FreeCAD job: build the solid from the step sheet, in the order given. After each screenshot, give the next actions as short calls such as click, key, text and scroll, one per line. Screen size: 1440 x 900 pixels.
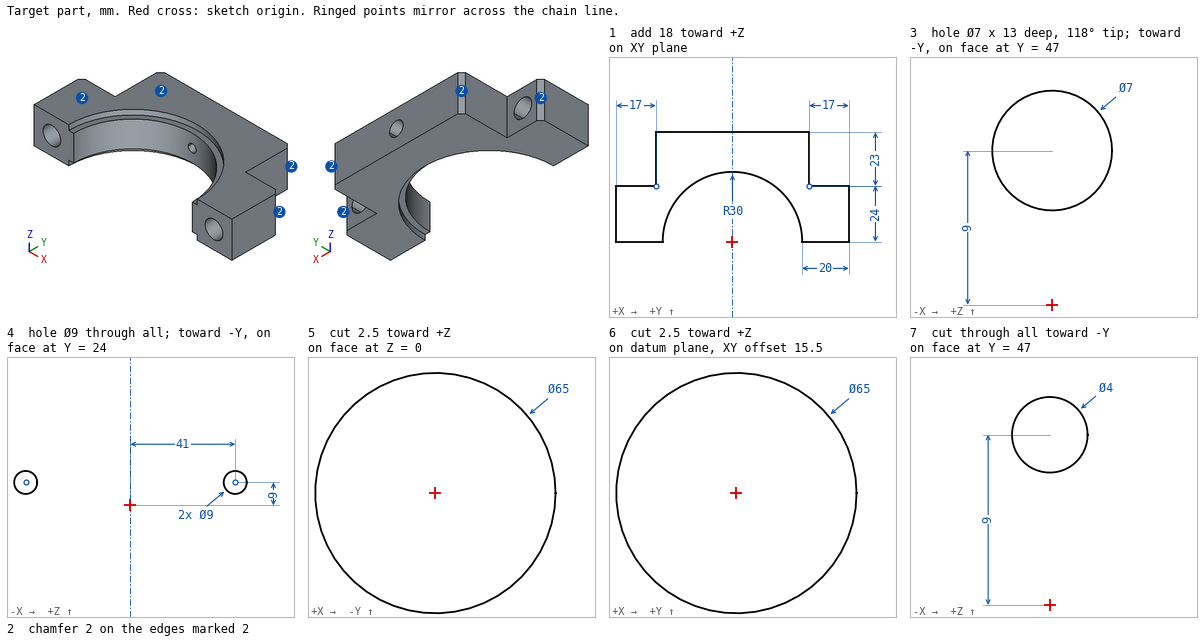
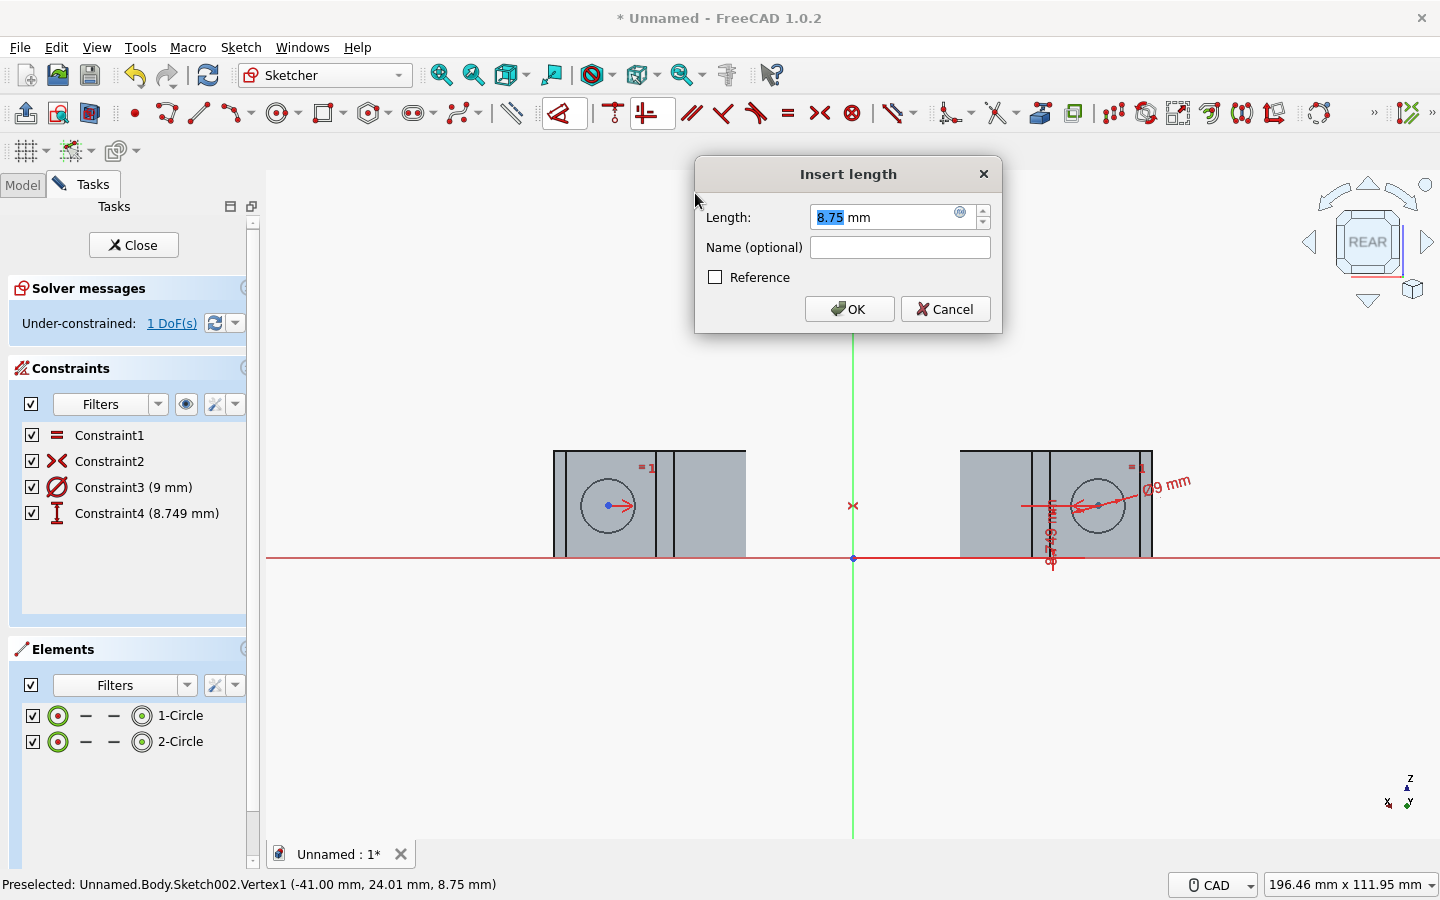
text(9)
key(Return)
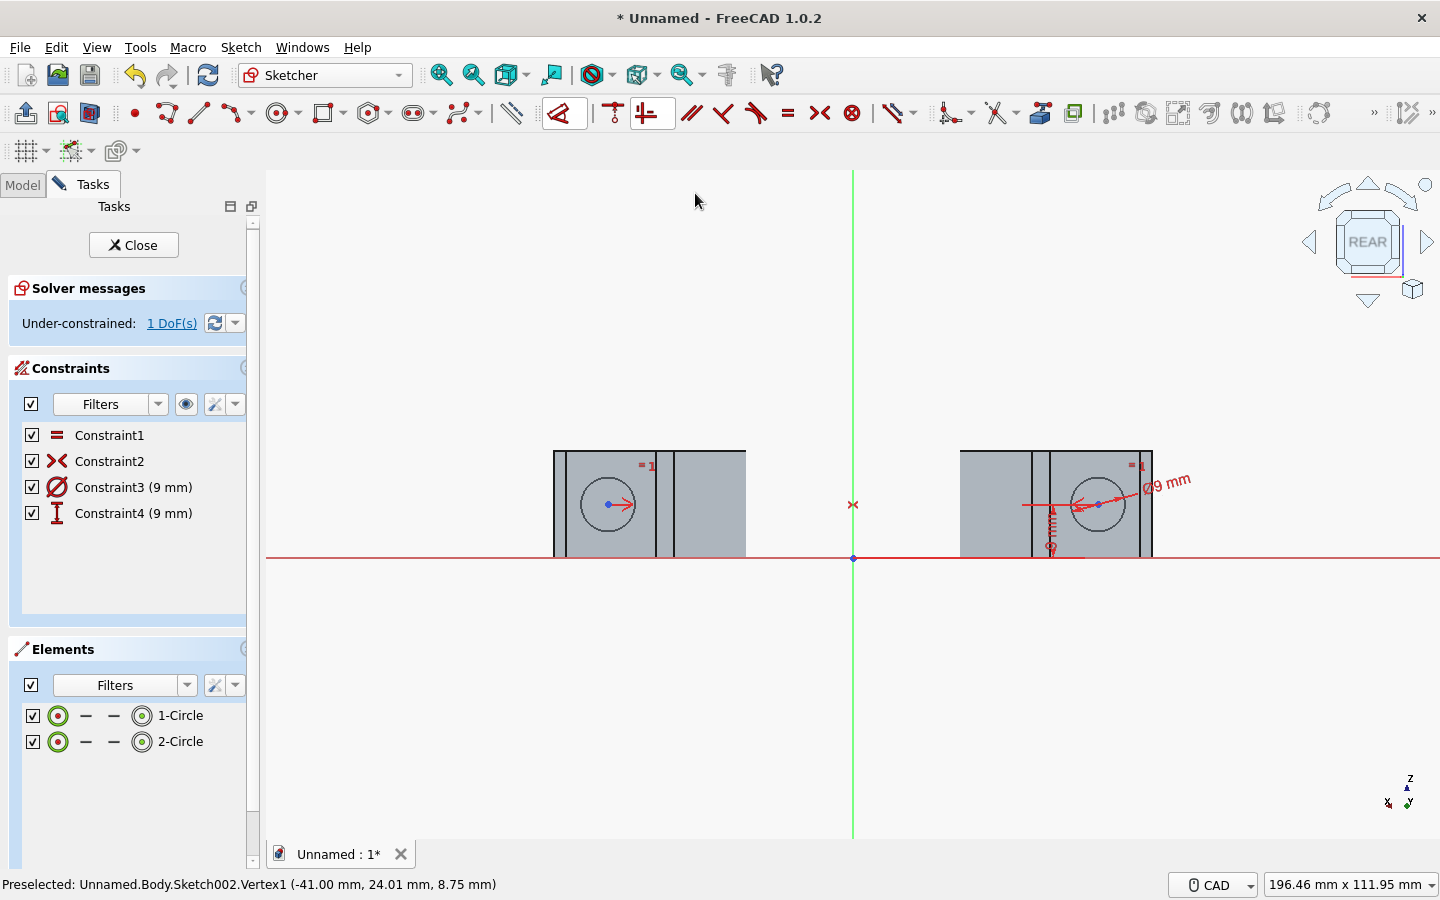
click(1098, 505)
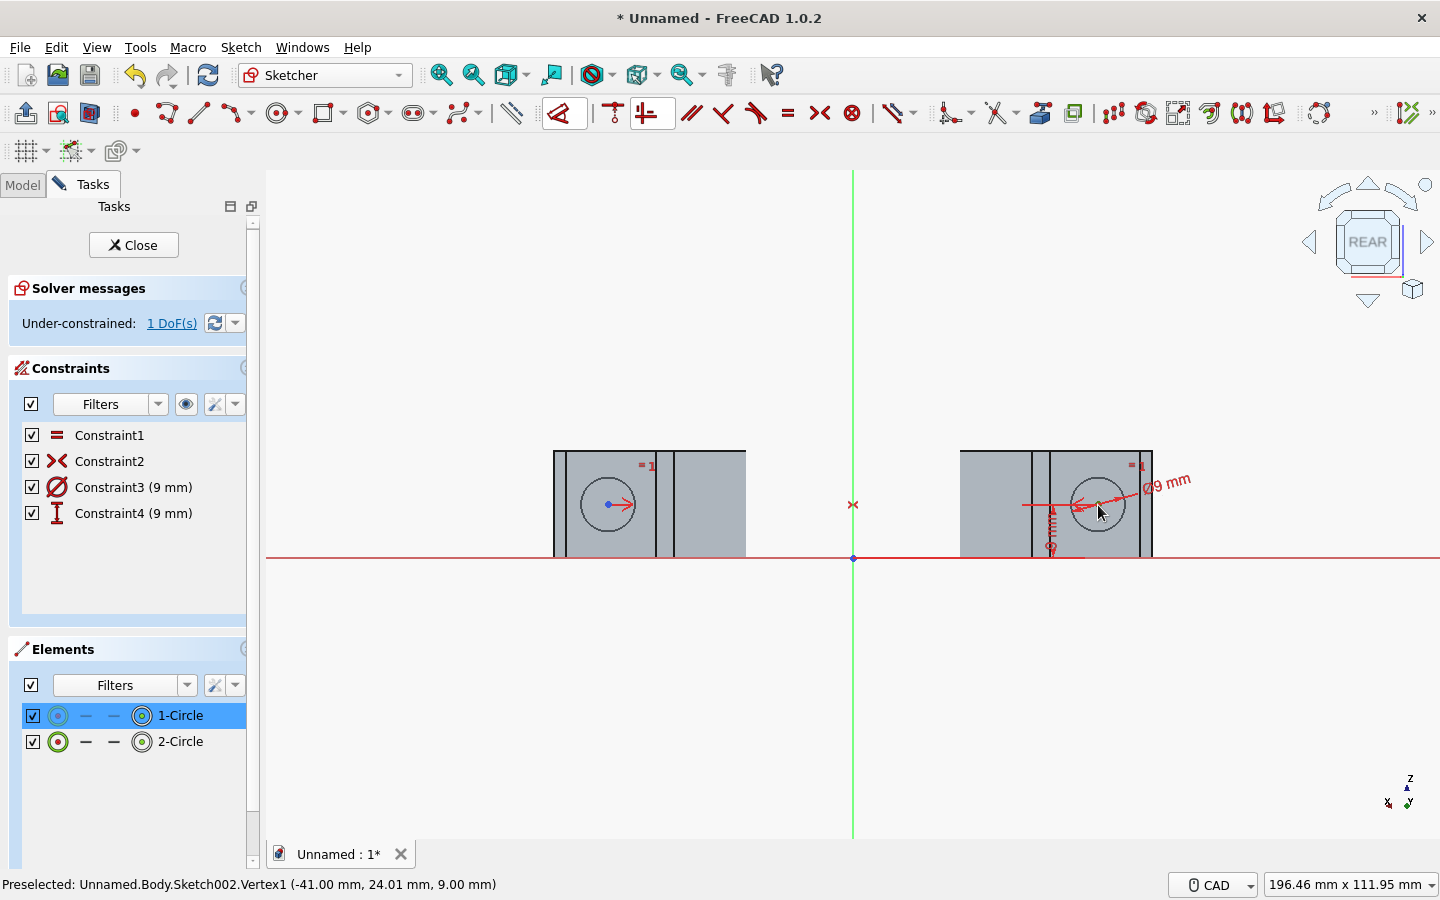
key(l)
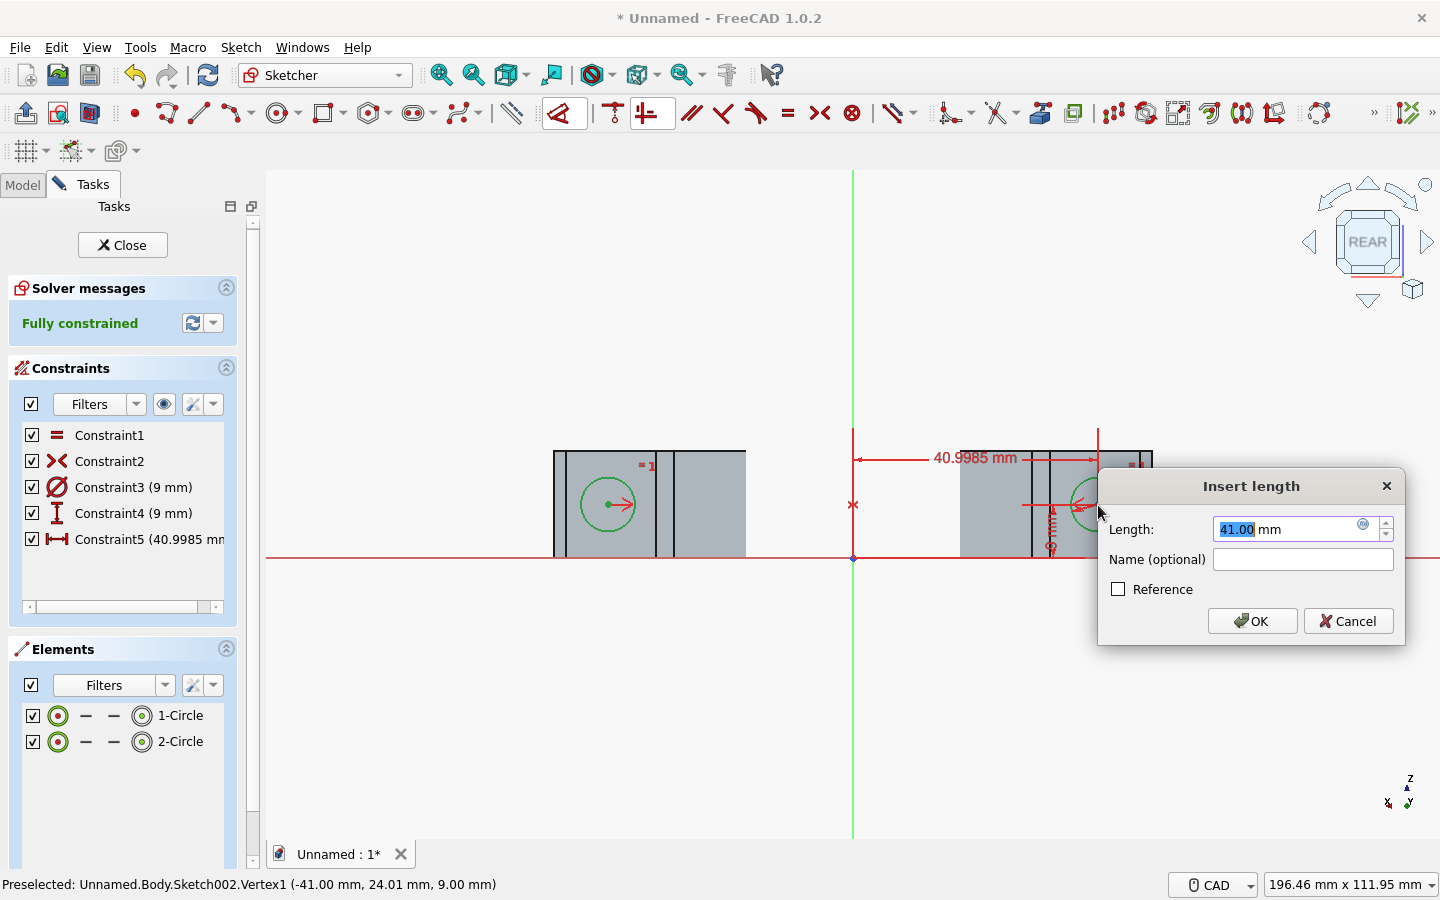
text(41)
key(Return)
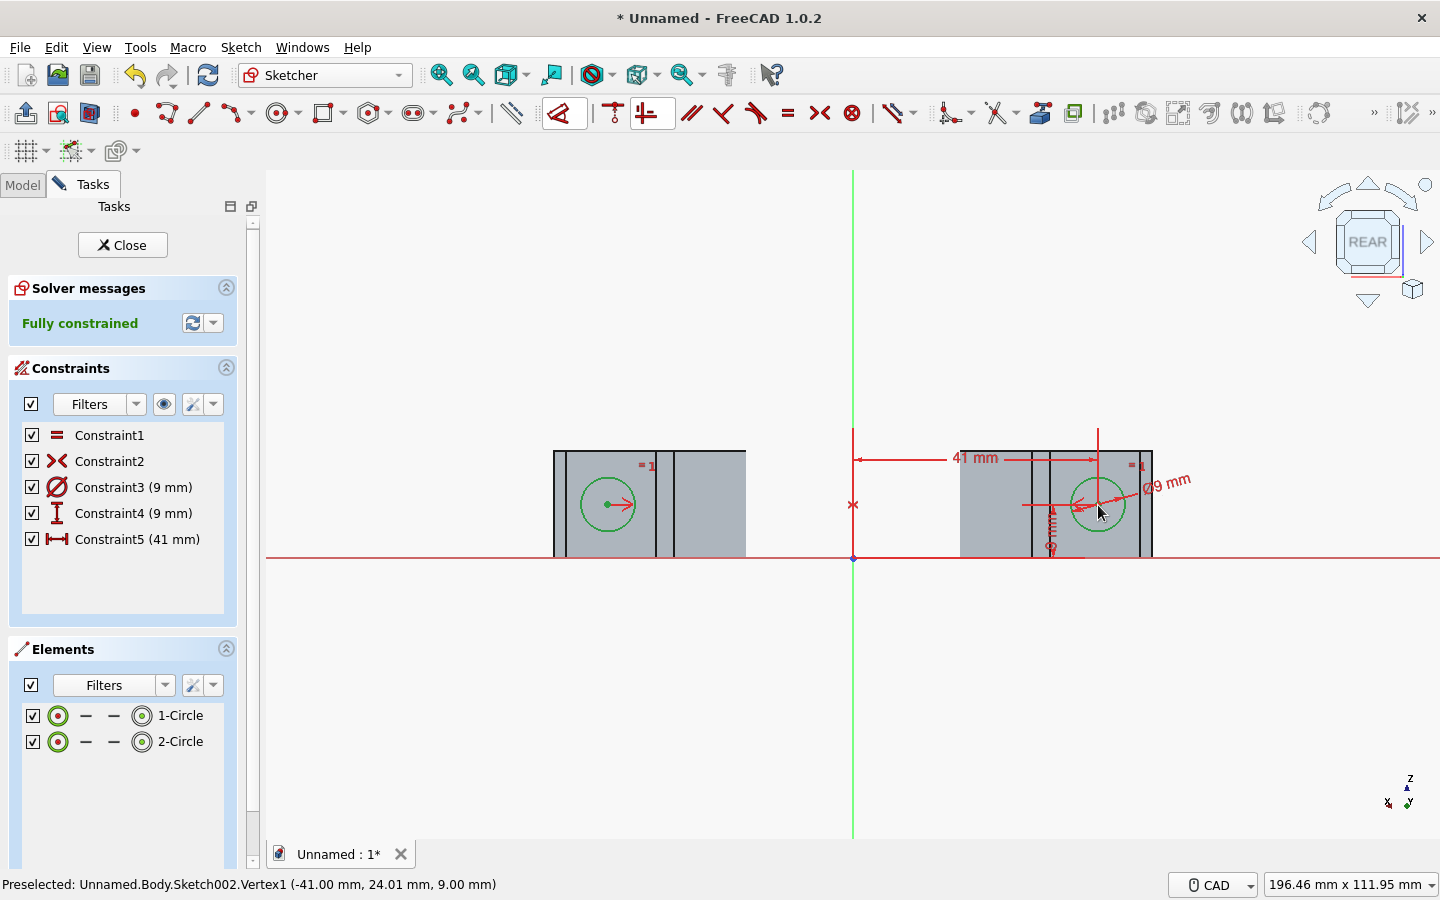
click(123, 245)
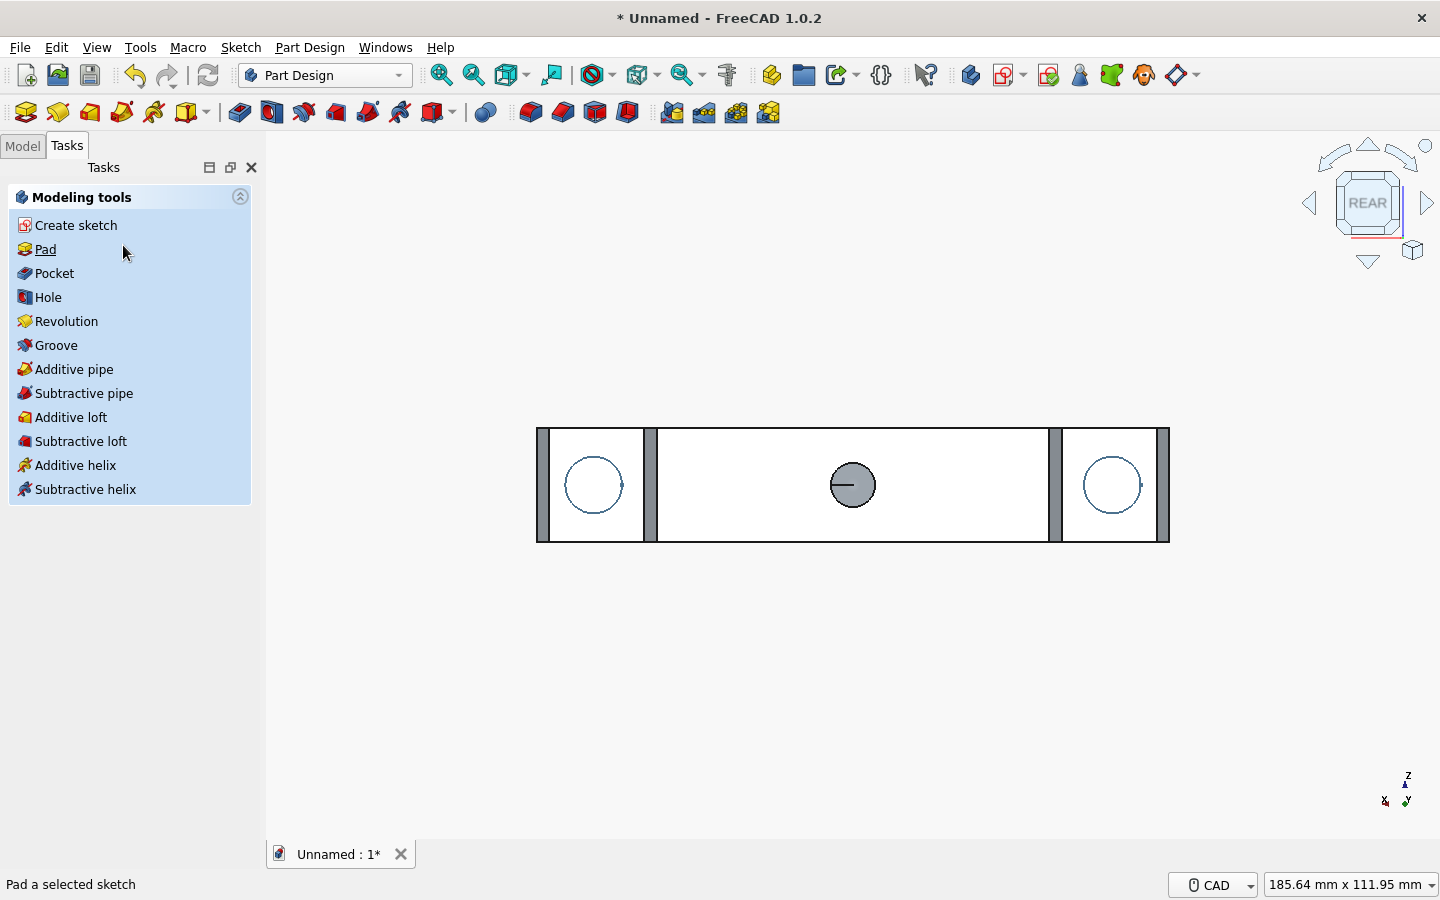
click(272, 112)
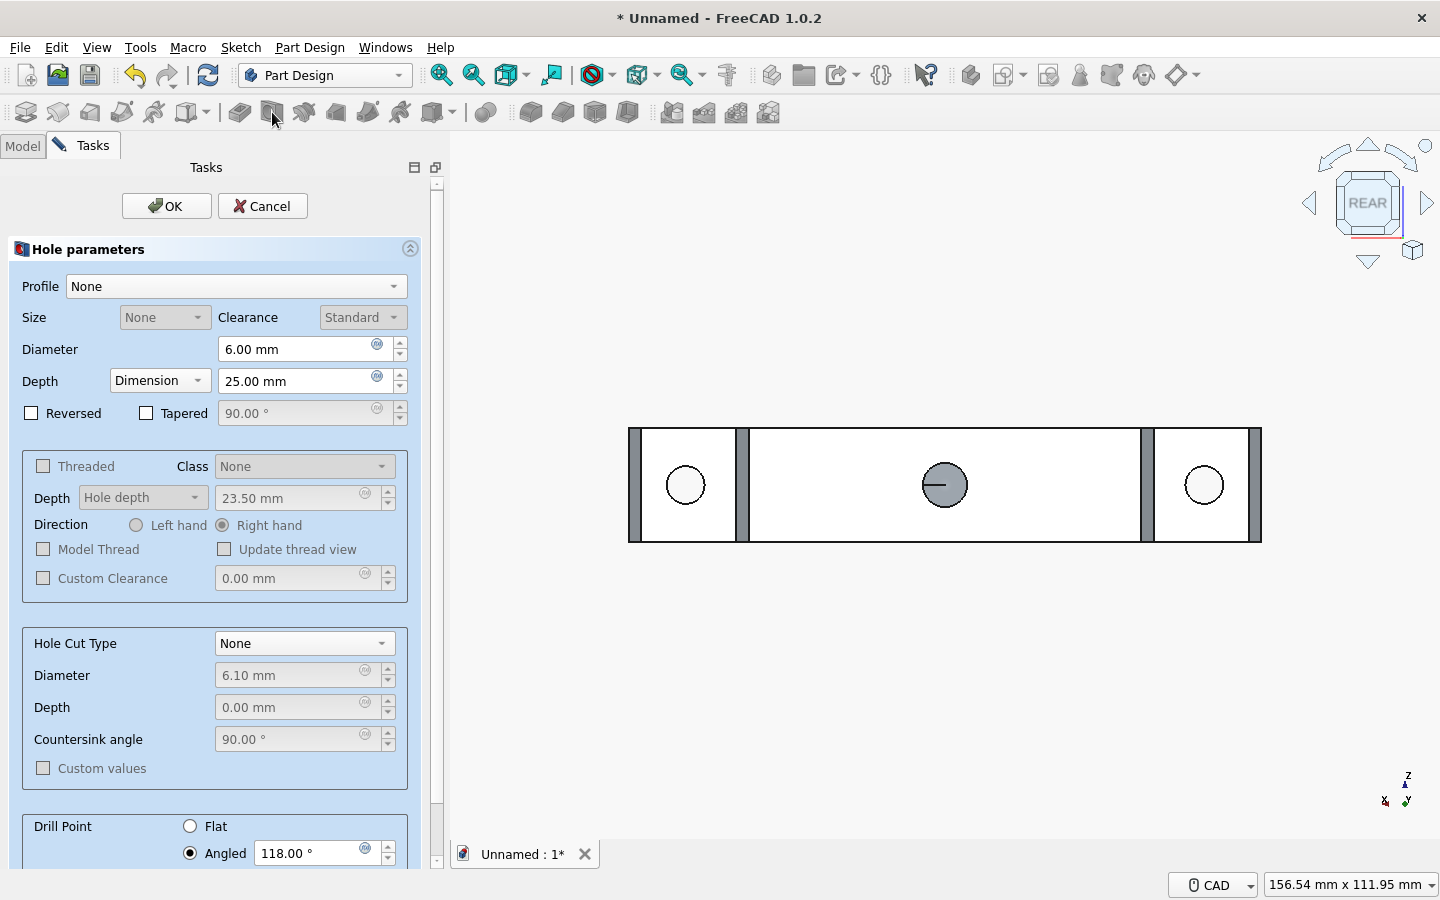
triple_click(305, 349)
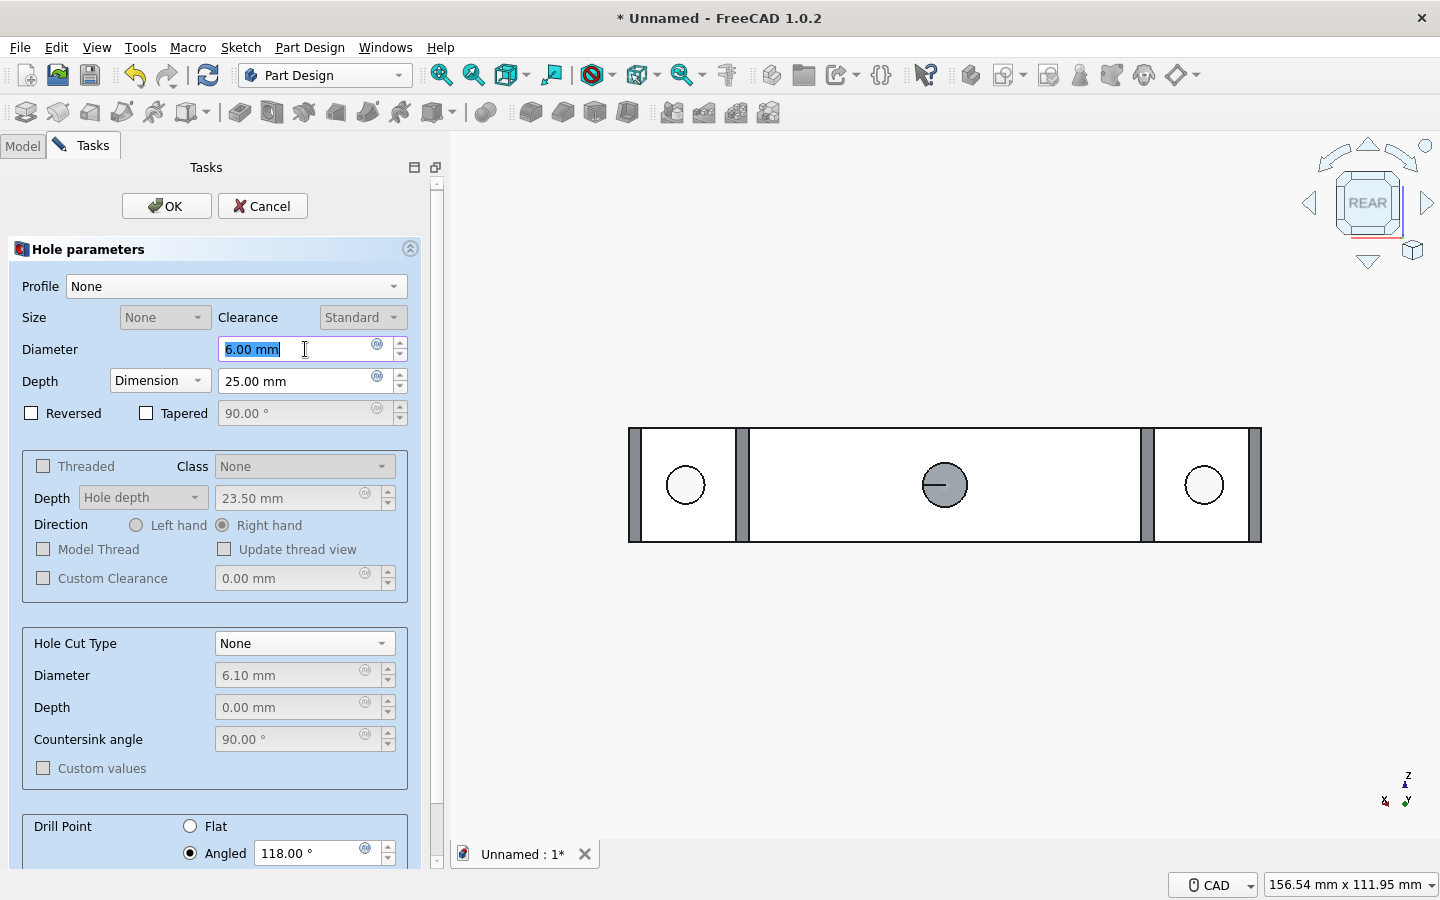
text(9)
key(Tab)